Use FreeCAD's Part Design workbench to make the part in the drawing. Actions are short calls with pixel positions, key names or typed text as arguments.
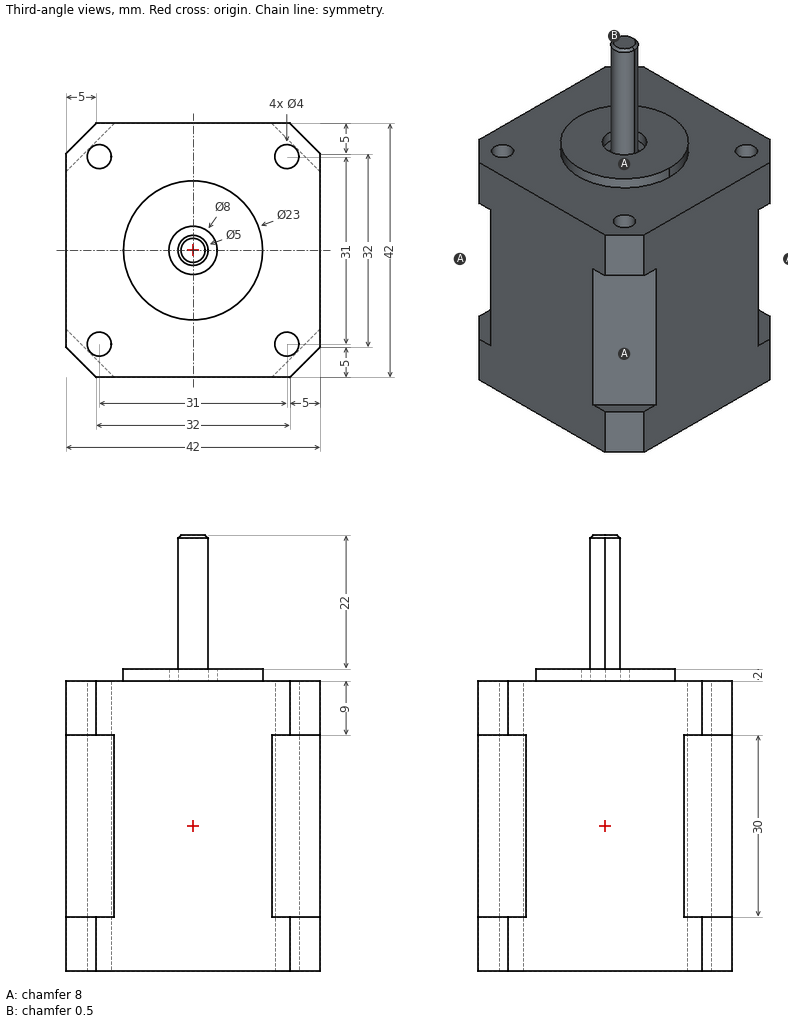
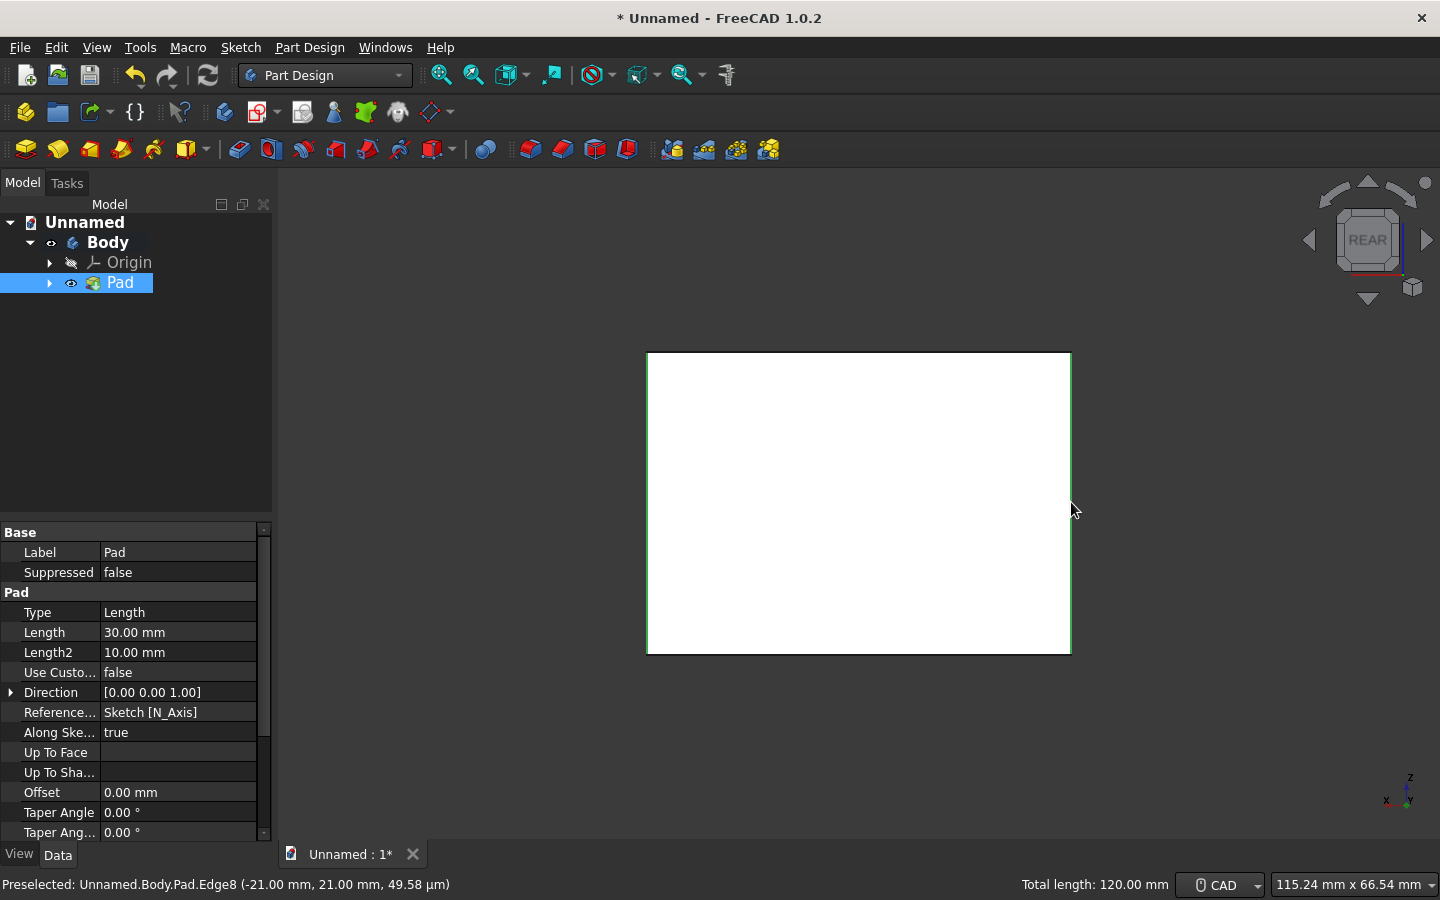
click(564, 150)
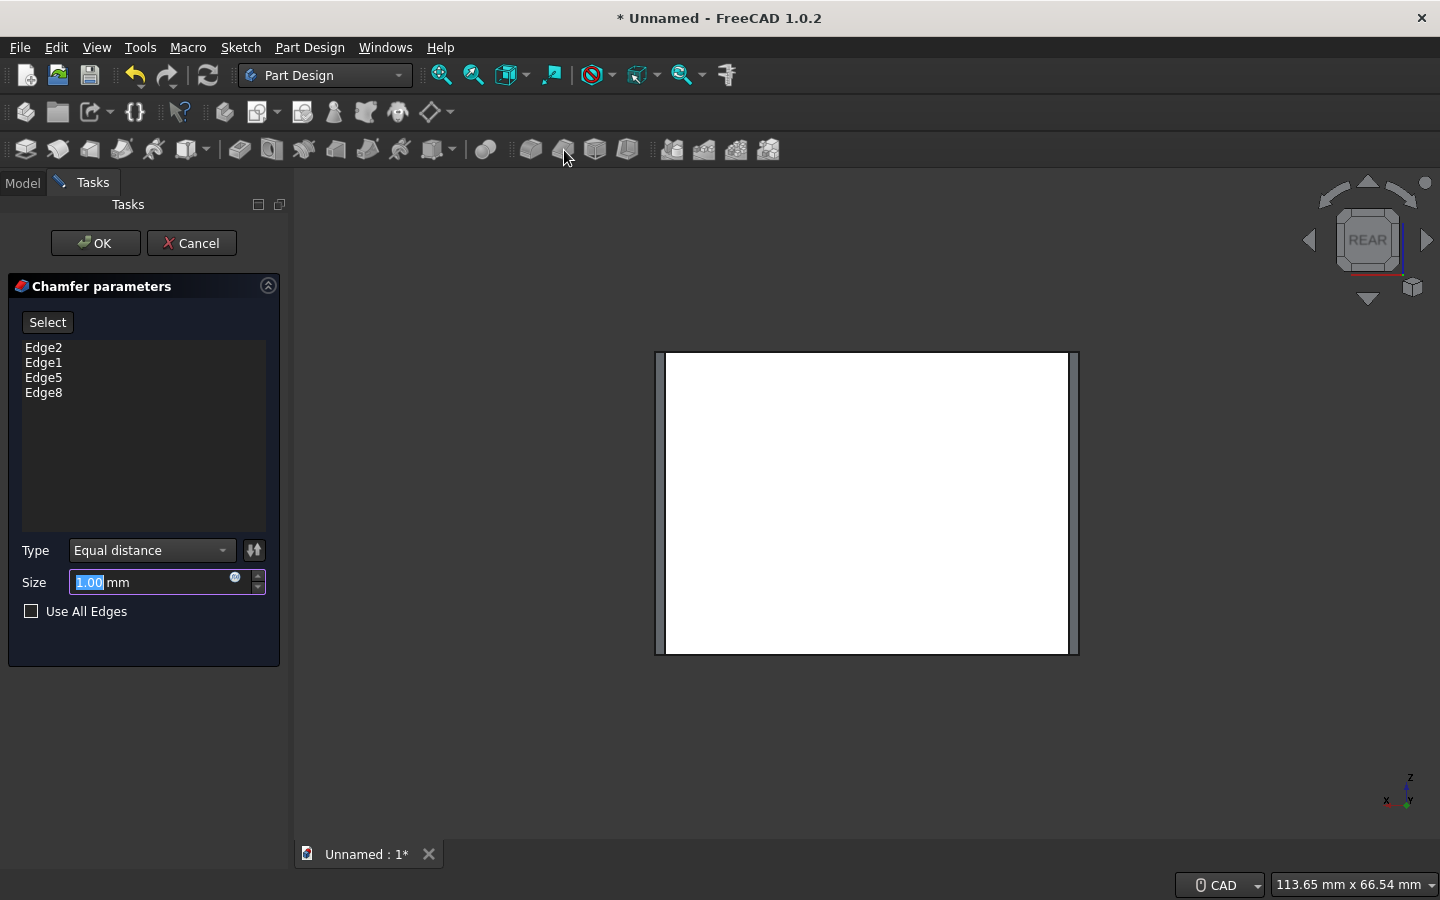
text(8)
key(Tab)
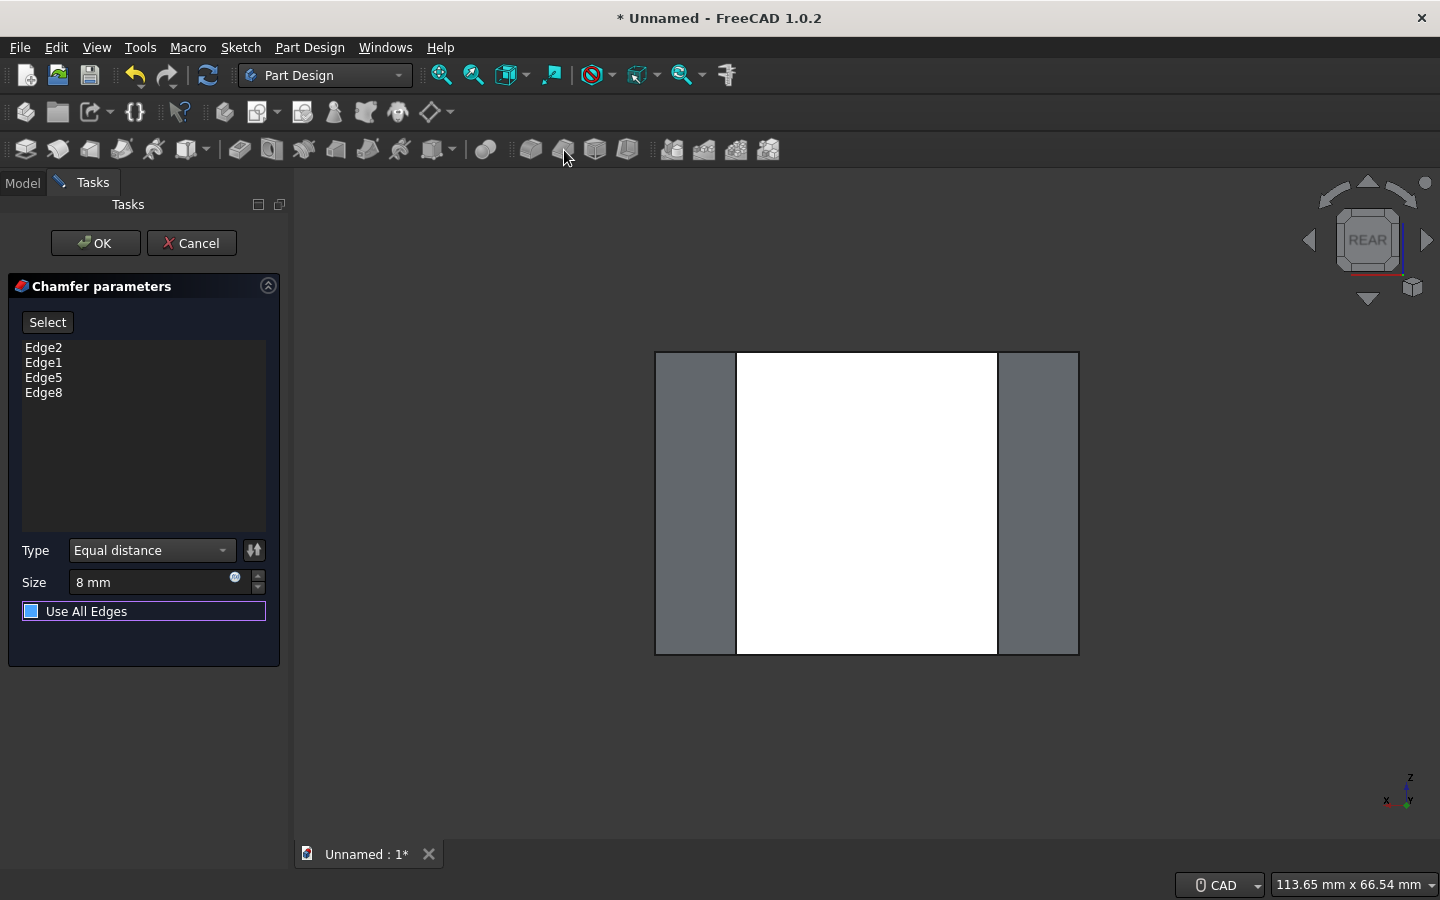
click(96, 243)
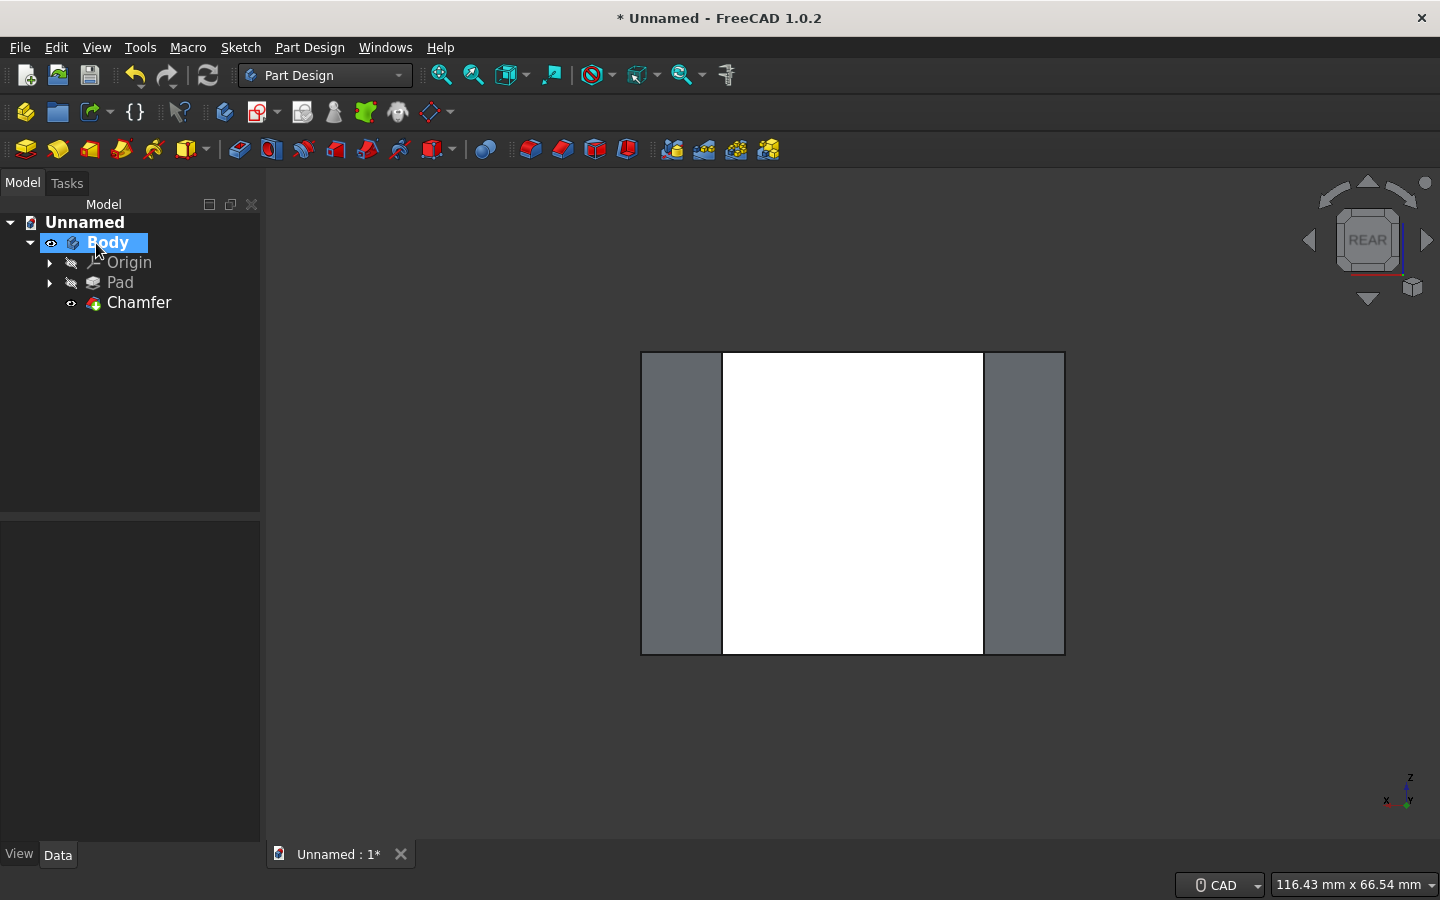
key(0)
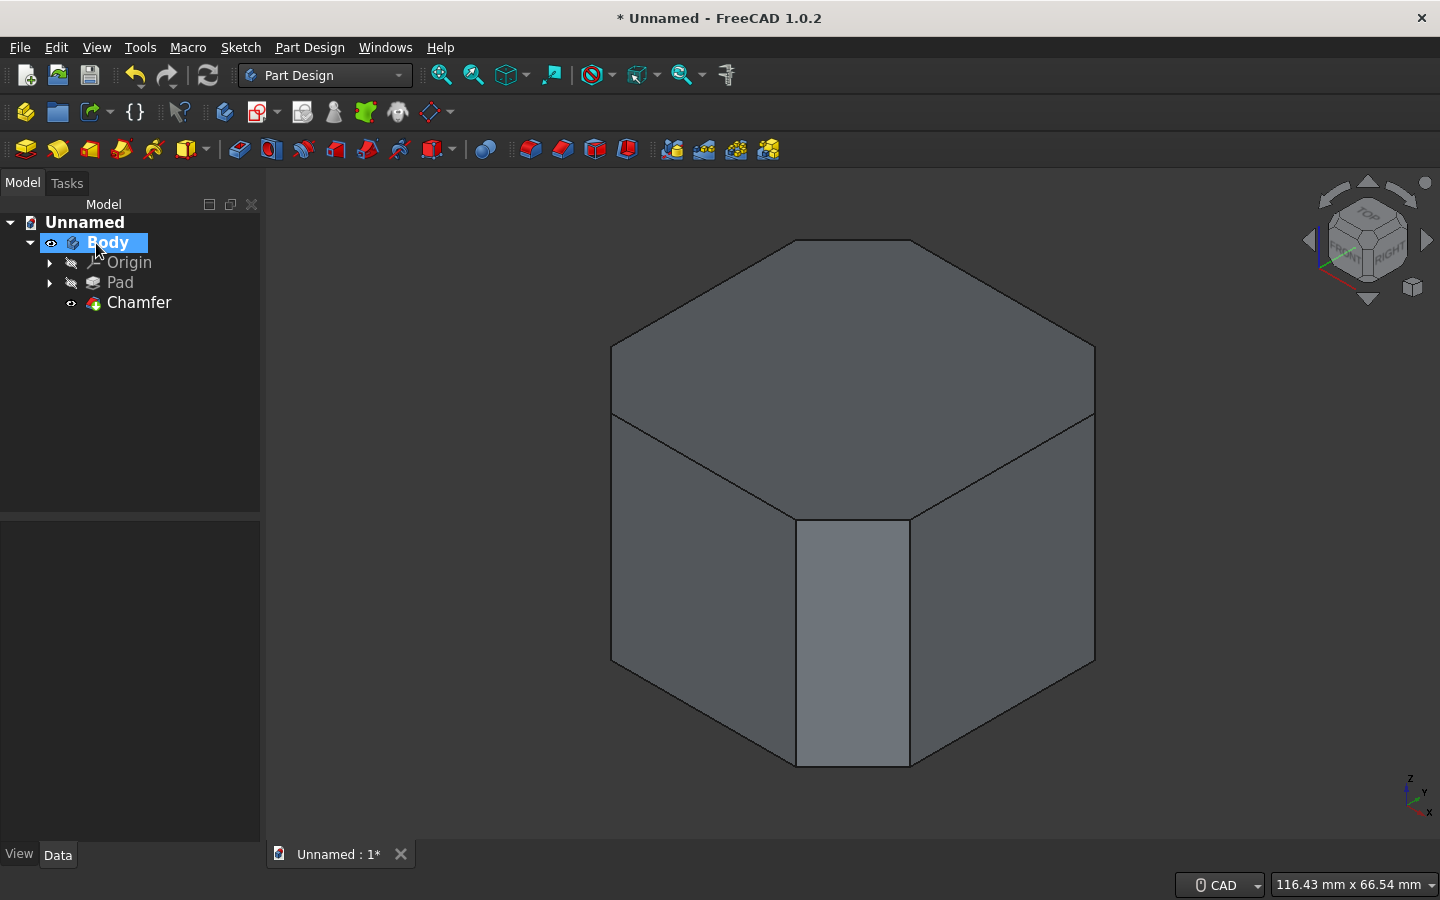
click(853, 379)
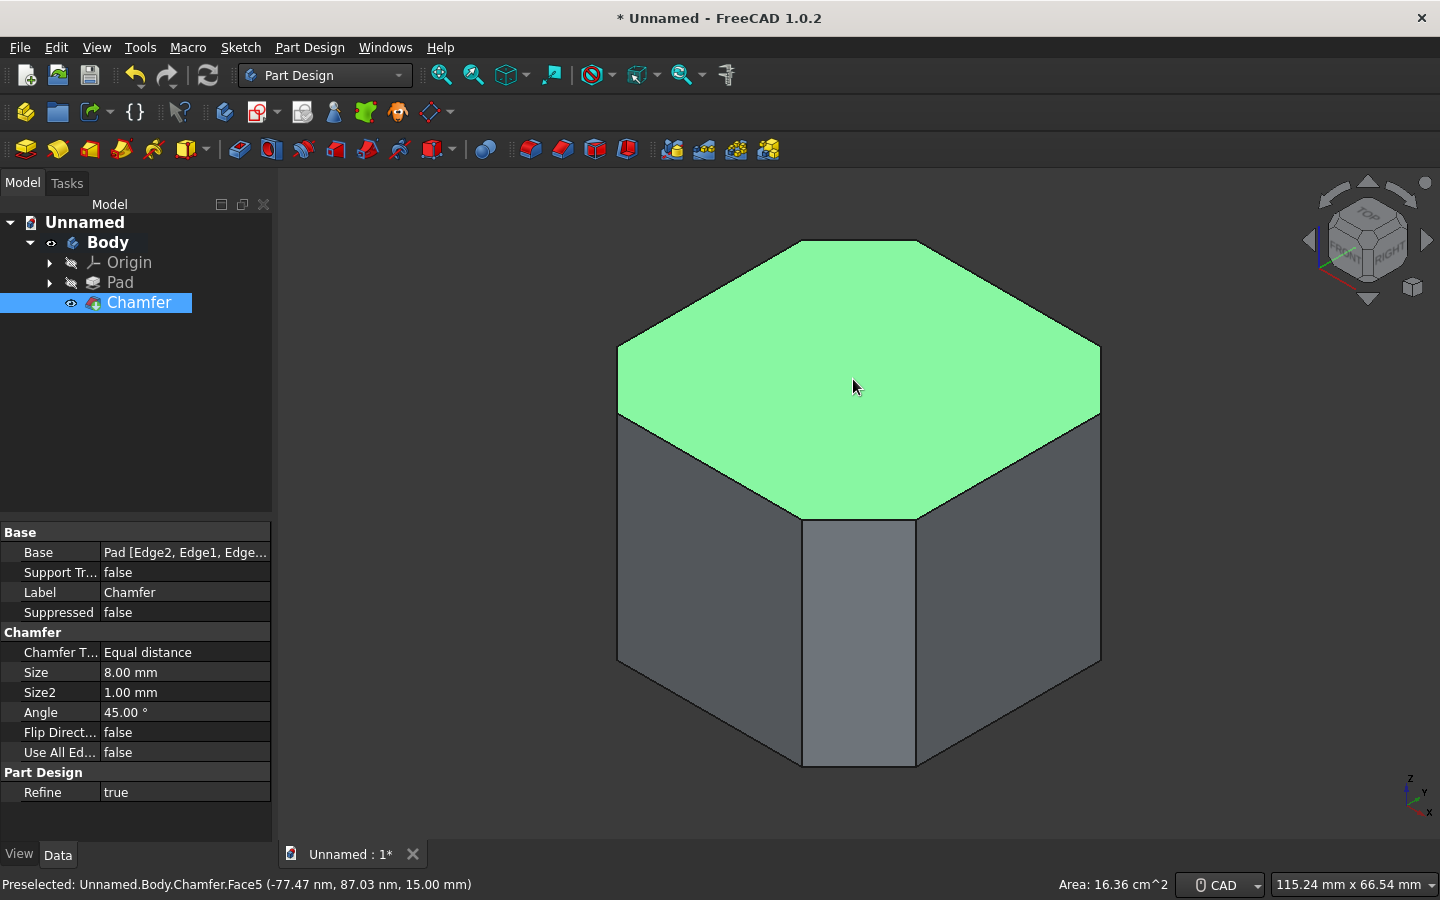
click(258, 112)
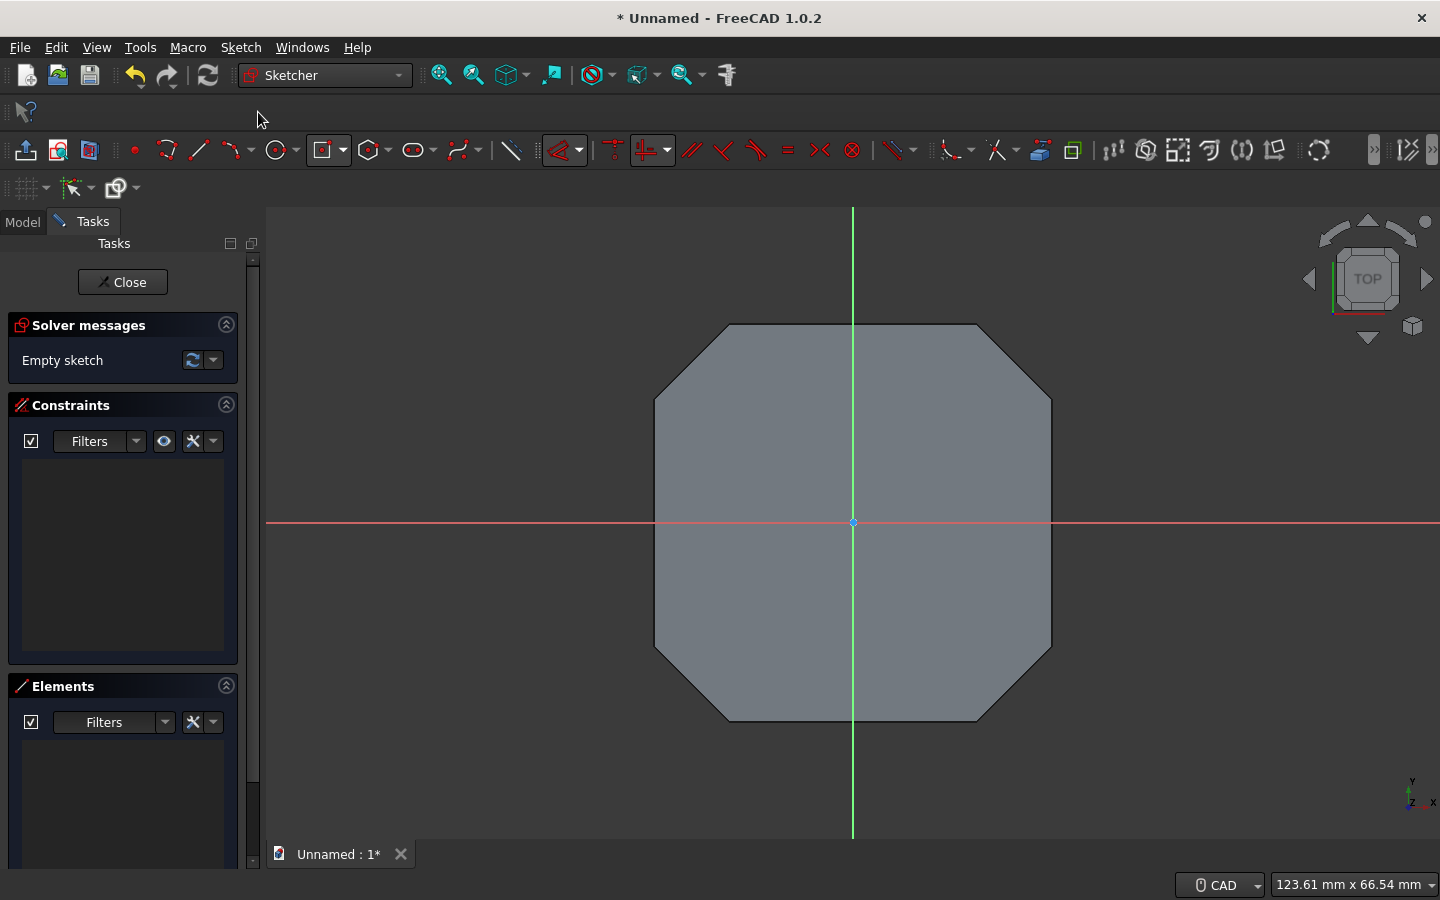
click(168, 150)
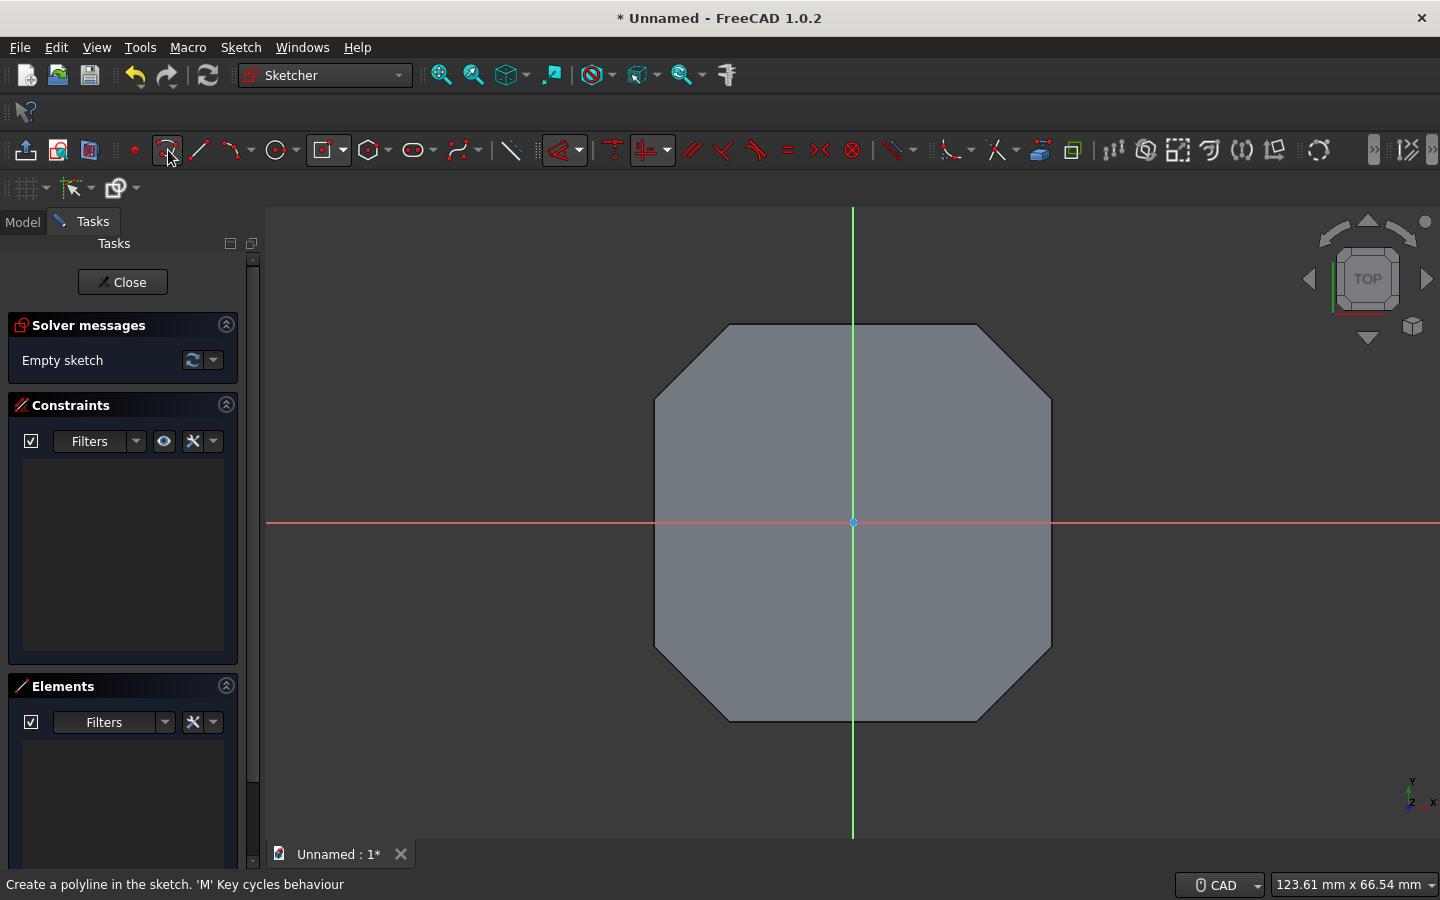
click(701, 722)
click(1005, 722)
click(1052, 675)
click(1052, 371)
click(1005, 324)
click(701, 324)
click(654, 371)
click(654, 675)
click(701, 723)
key(Escape)
key(Escape)